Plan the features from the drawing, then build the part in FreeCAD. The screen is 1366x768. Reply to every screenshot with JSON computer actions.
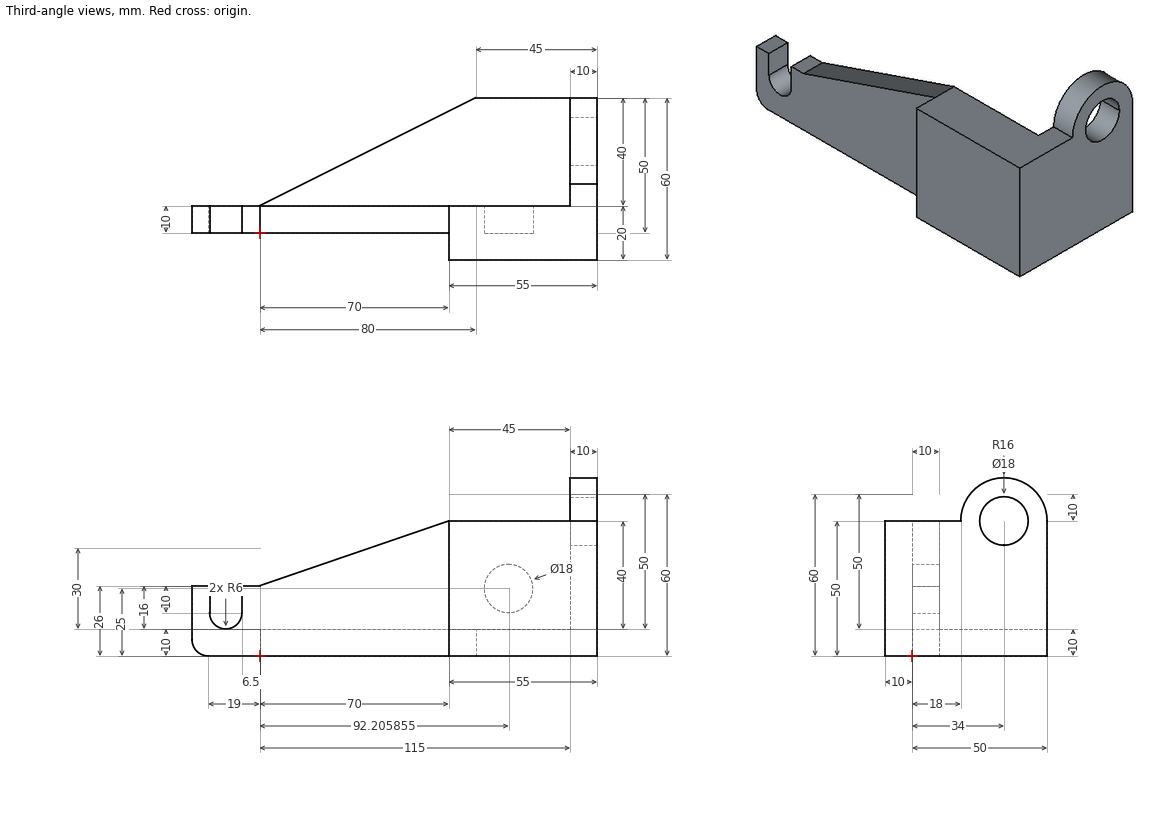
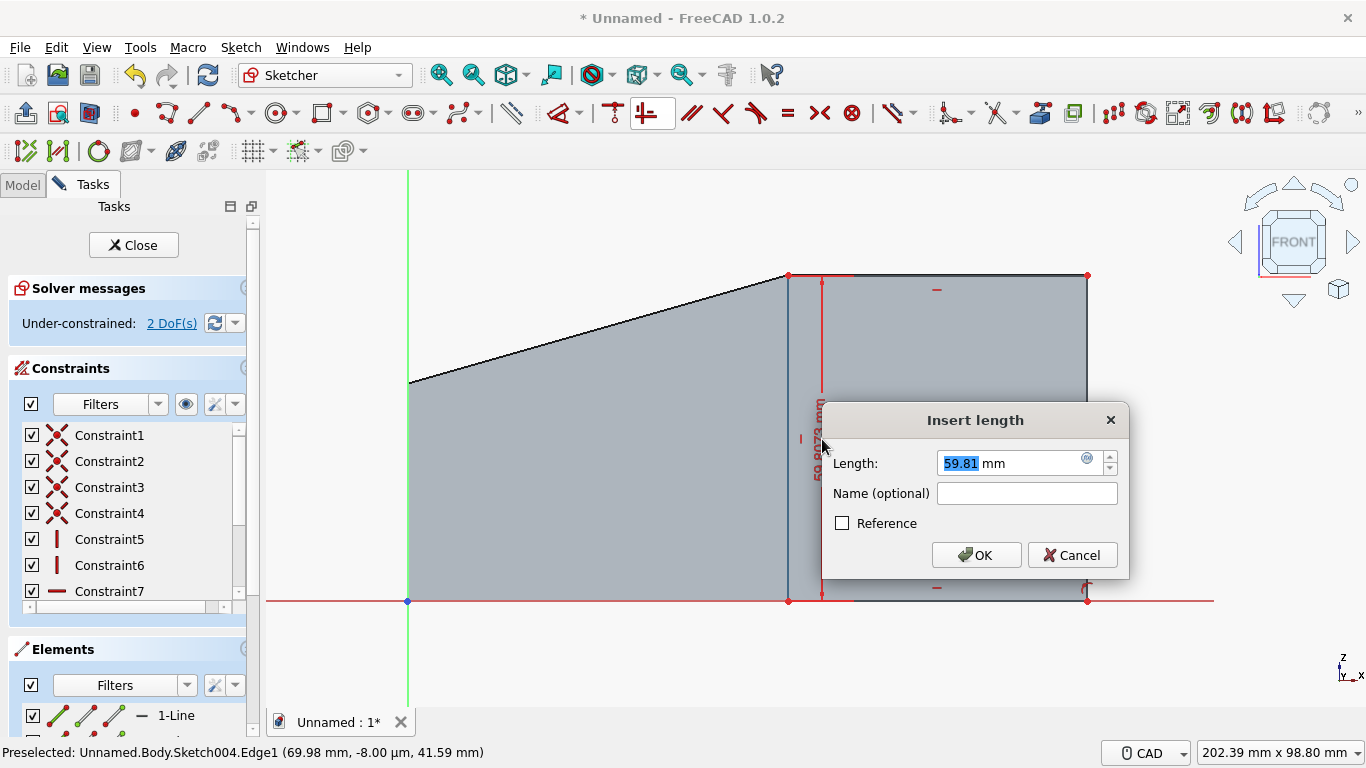
{"action": "type", "text": "60"}
{"action": "key", "text": "Return"}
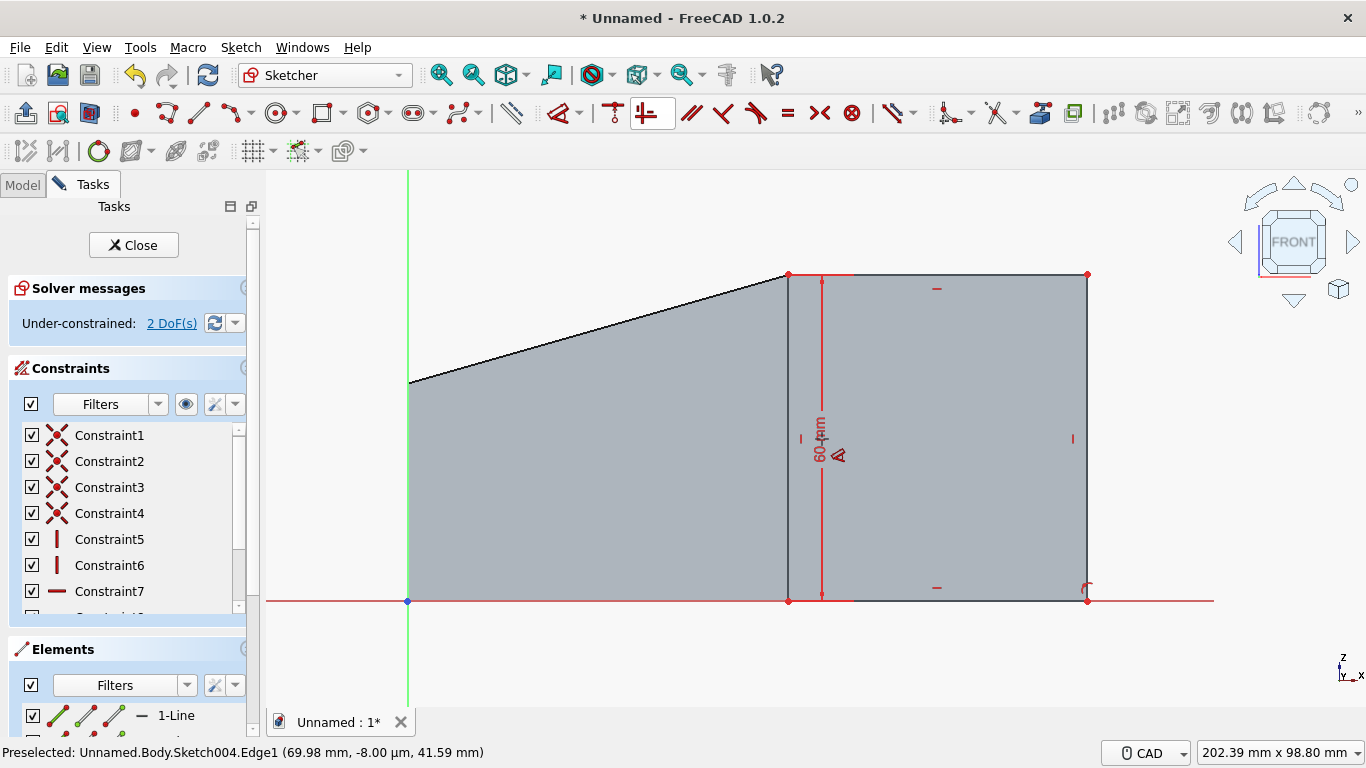
{"action": "left_click", "coordinate": [878, 601]}
{"action": "left_click", "coordinate": [937, 635]}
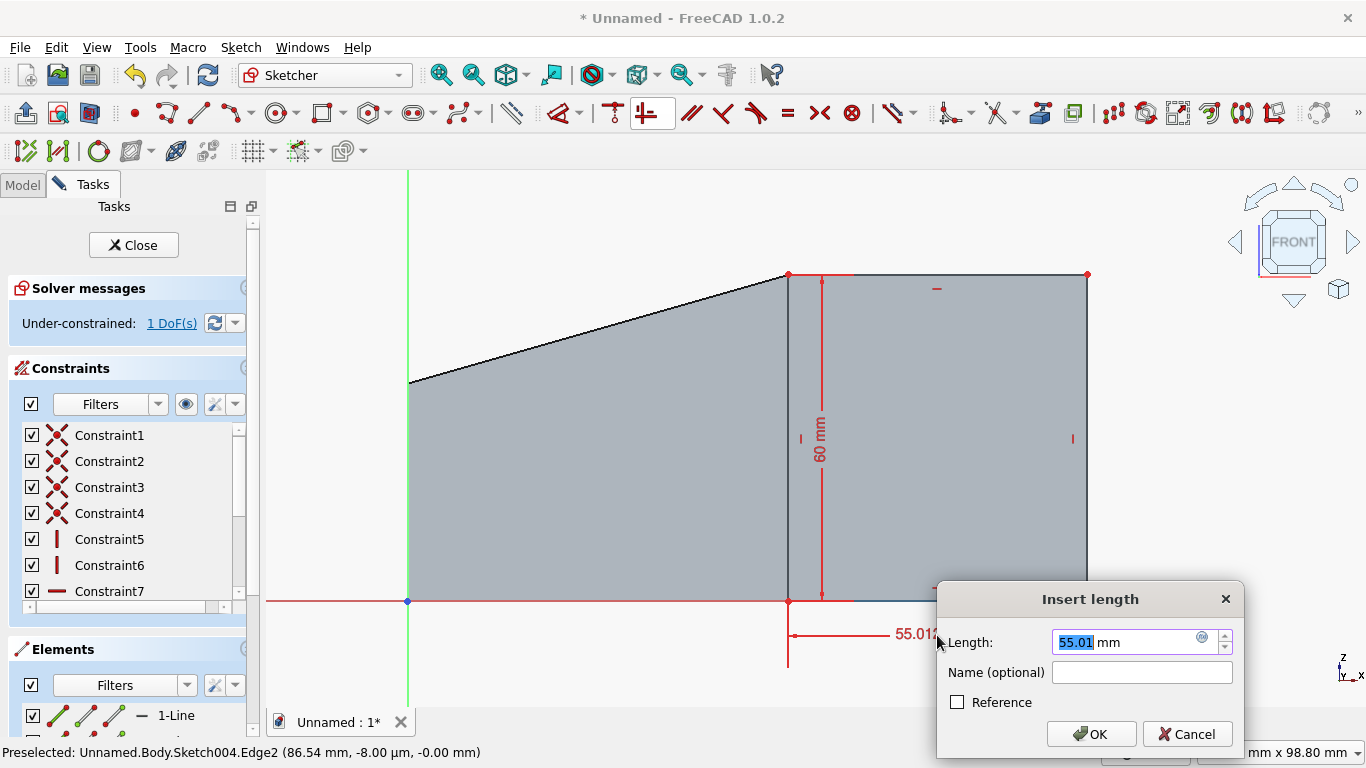
{"action": "type", "text": "55"}
{"action": "key", "text": "Return"}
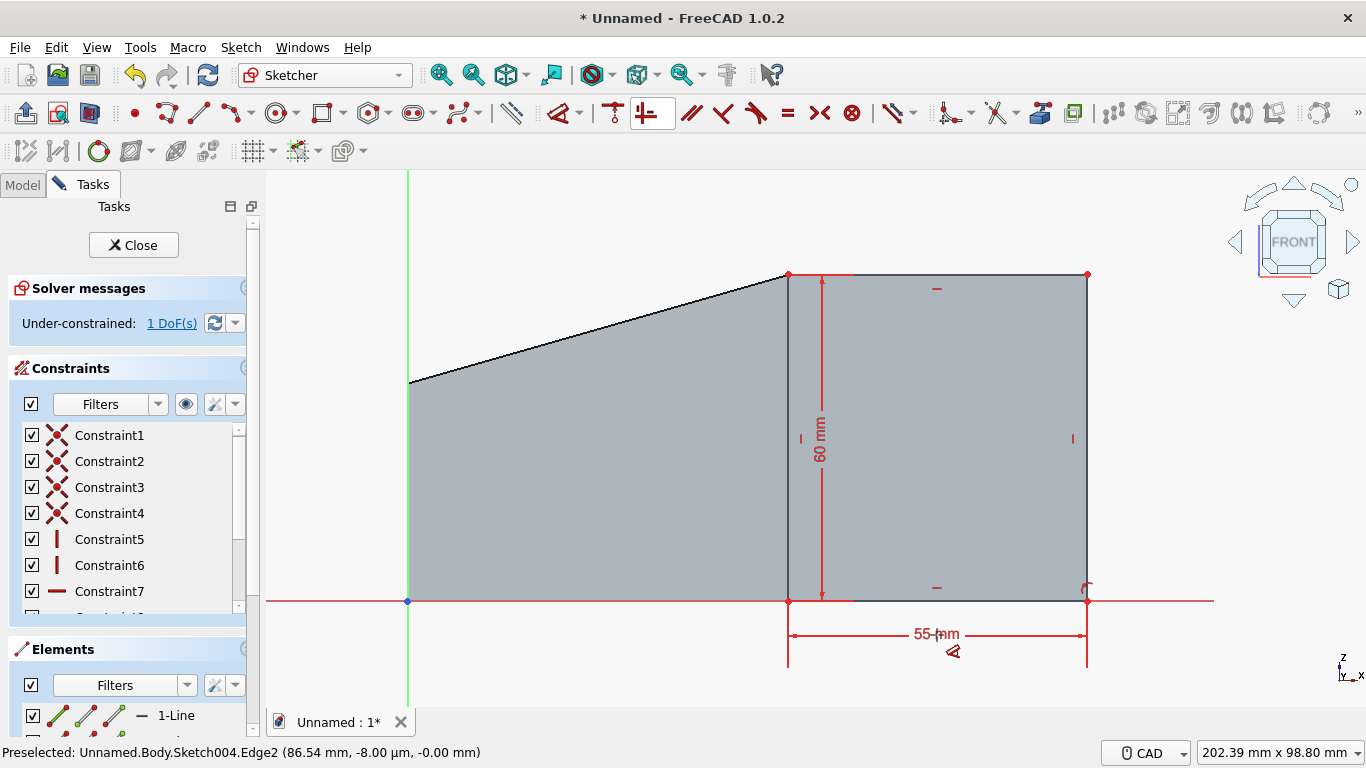
{"action": "left_click", "coordinate": [788, 275]}
{"action": "left_click", "coordinate": [598, 635]}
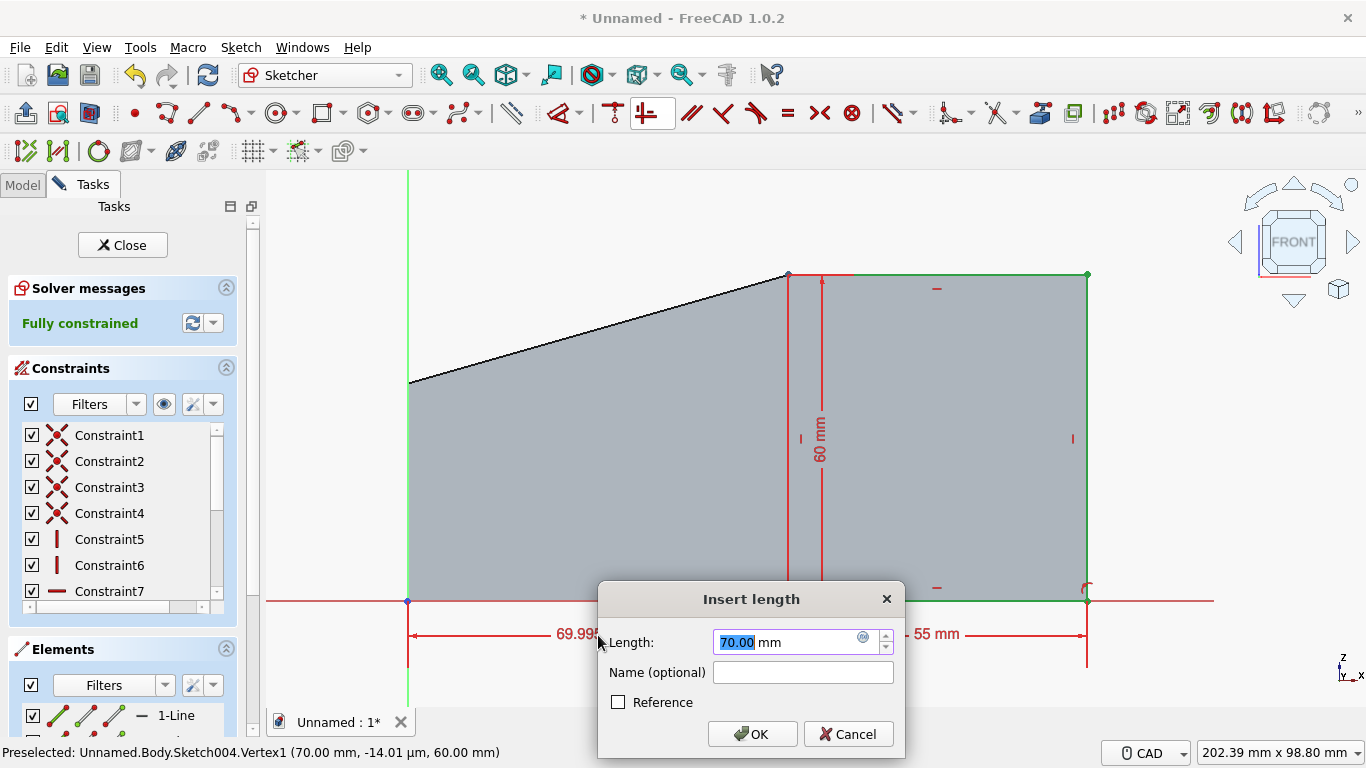
{"action": "type", "text": "70"}
{"action": "key", "text": "Return"}
{"action": "key", "text": "Escape"}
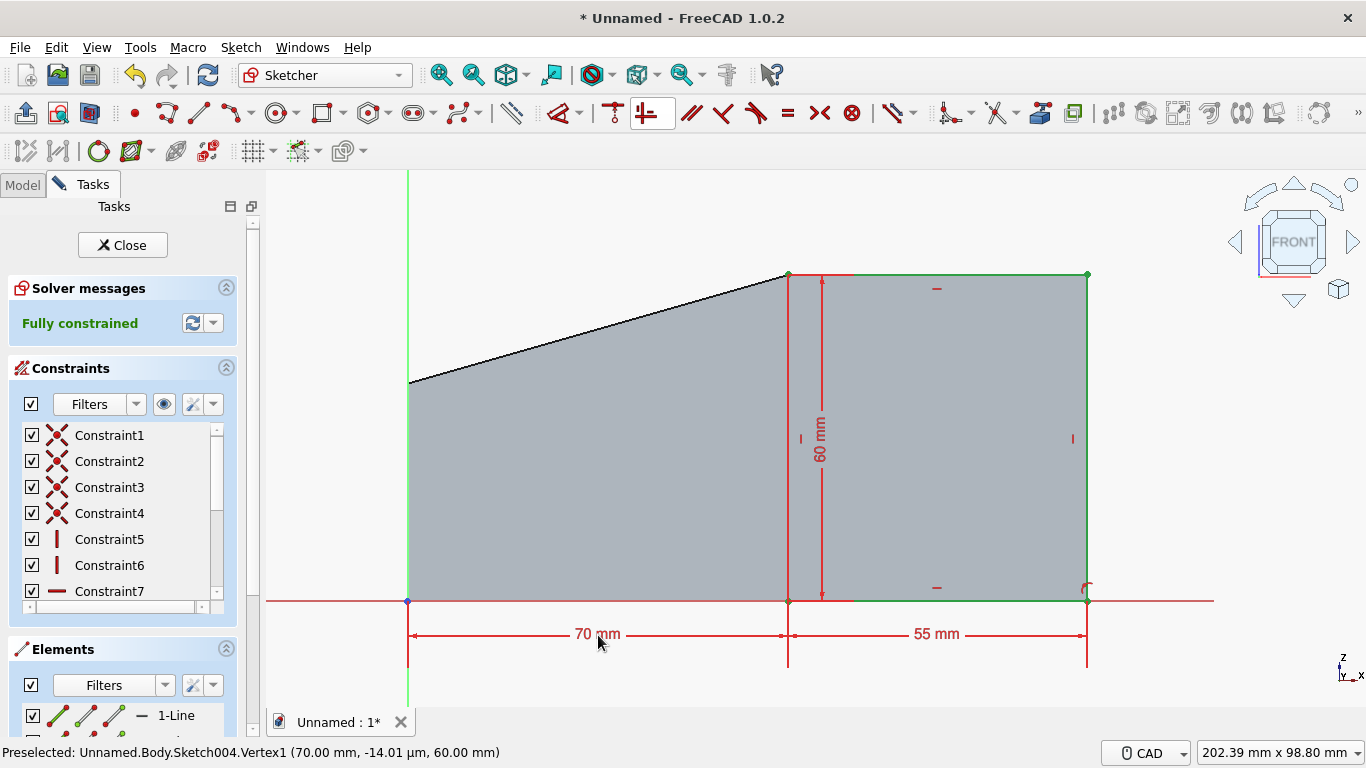
{"action": "left_click", "coordinate": [123, 245]}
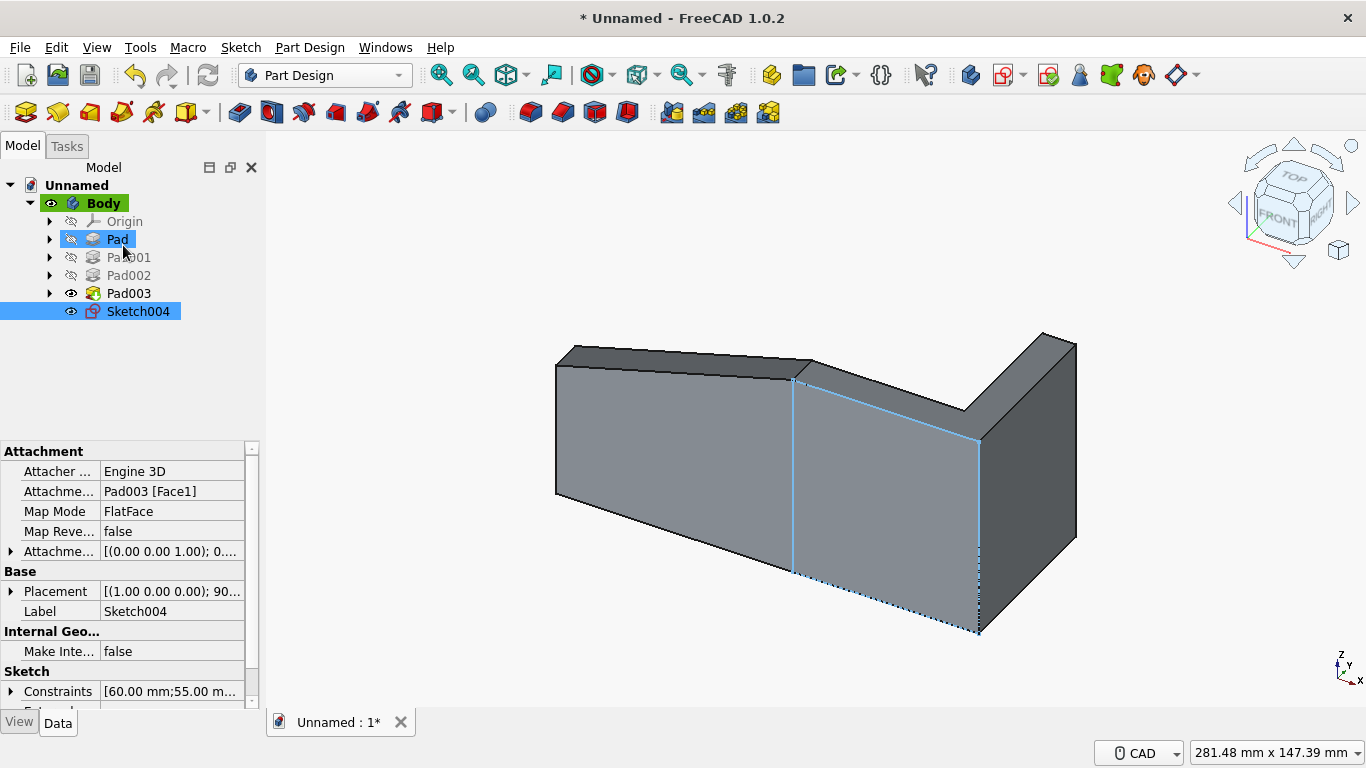
{"action": "left_click", "coordinate": [26, 112]}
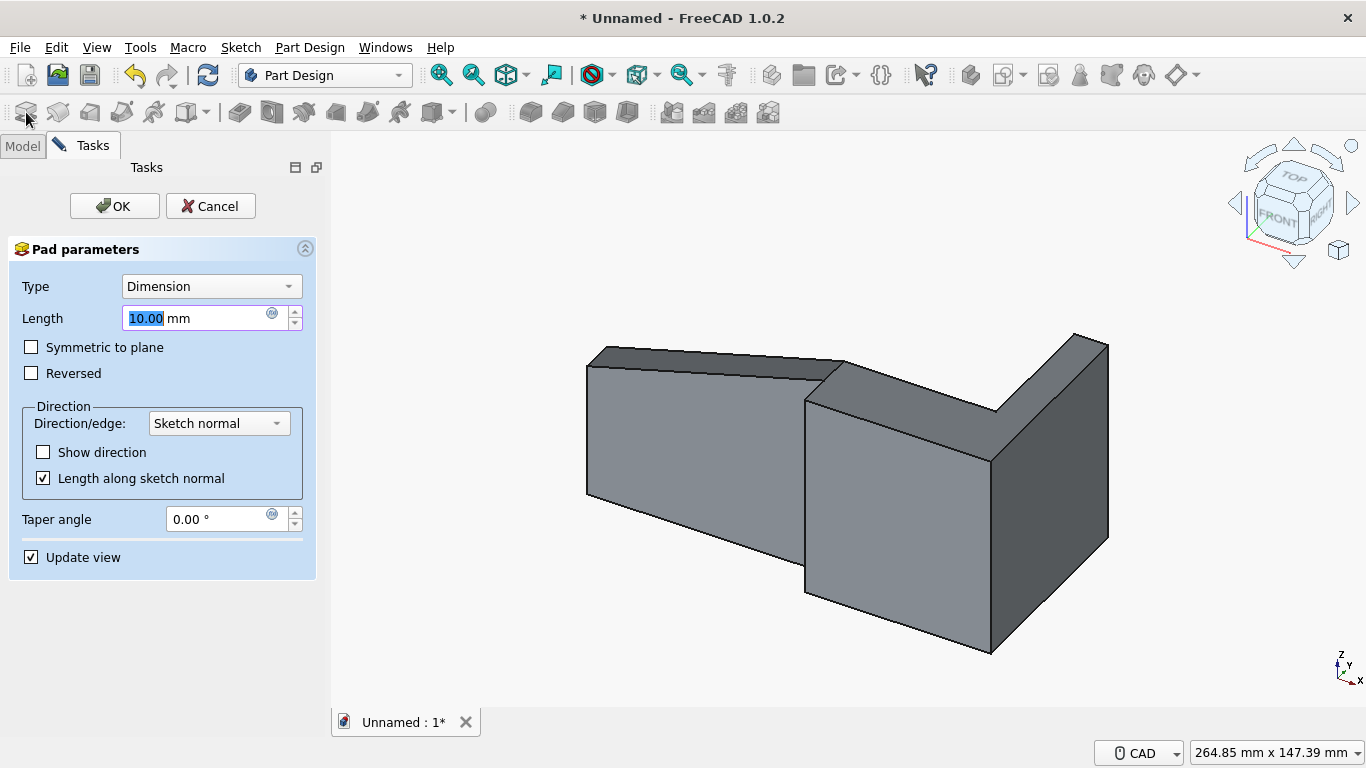
{"action": "type", "text": "10"}
{"action": "key", "text": "Tab"}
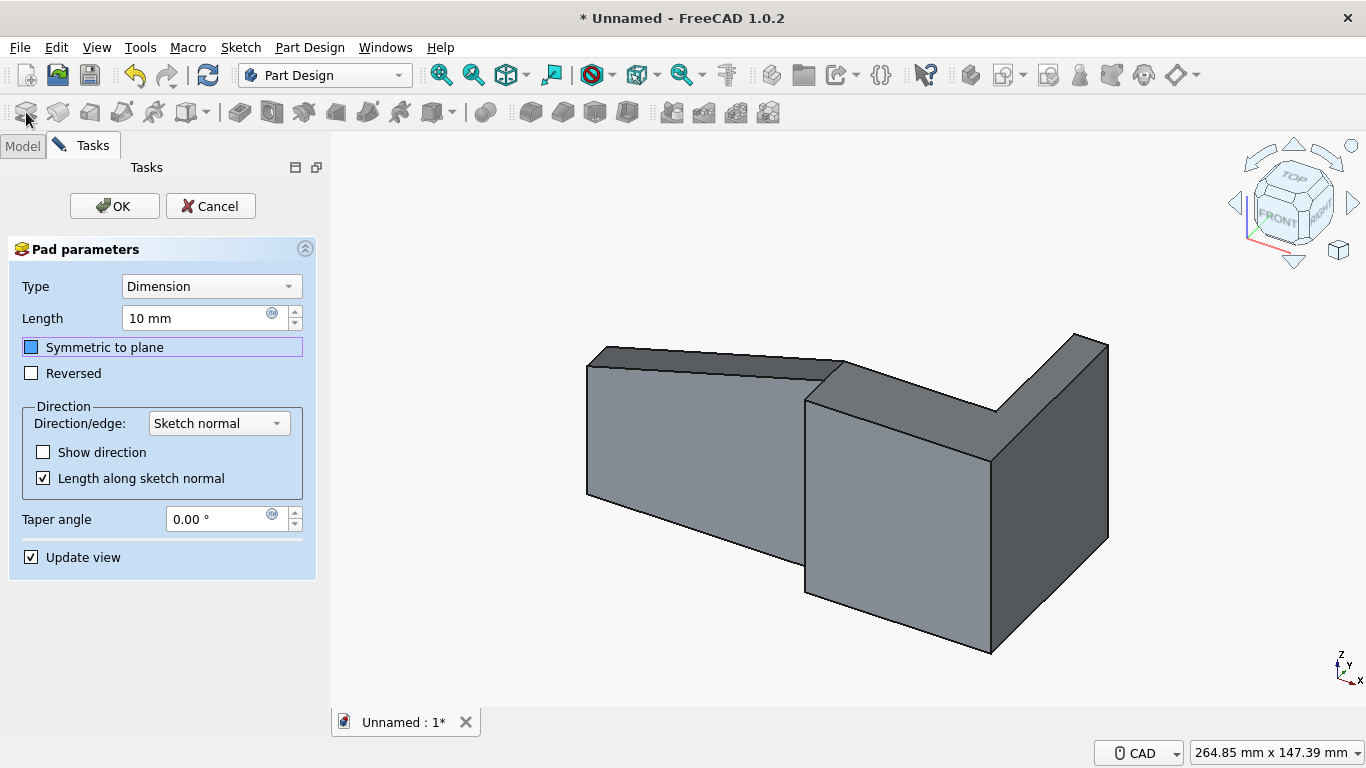
{"action": "left_click", "coordinate": [115, 206]}